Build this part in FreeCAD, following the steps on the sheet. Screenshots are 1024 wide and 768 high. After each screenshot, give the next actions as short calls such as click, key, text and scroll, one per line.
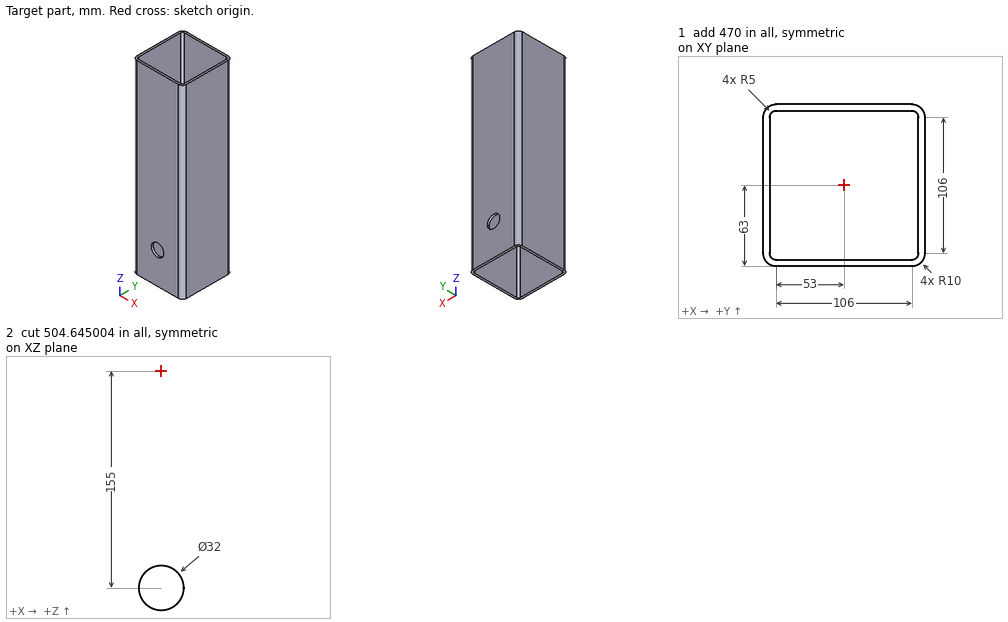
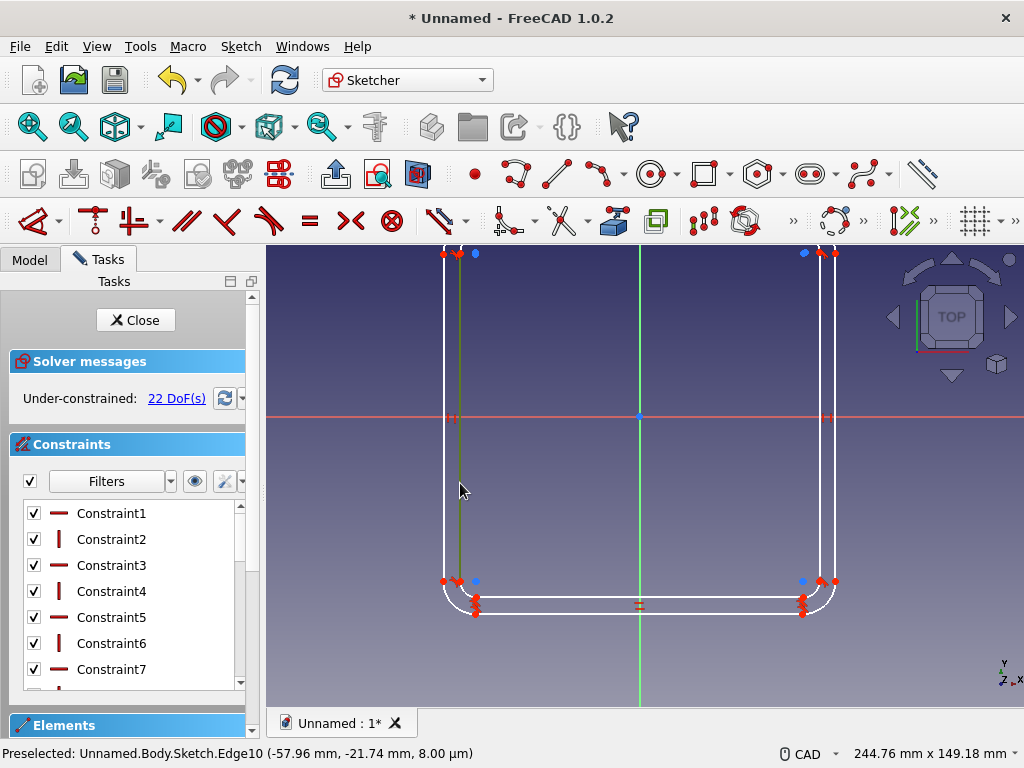
click(465, 593)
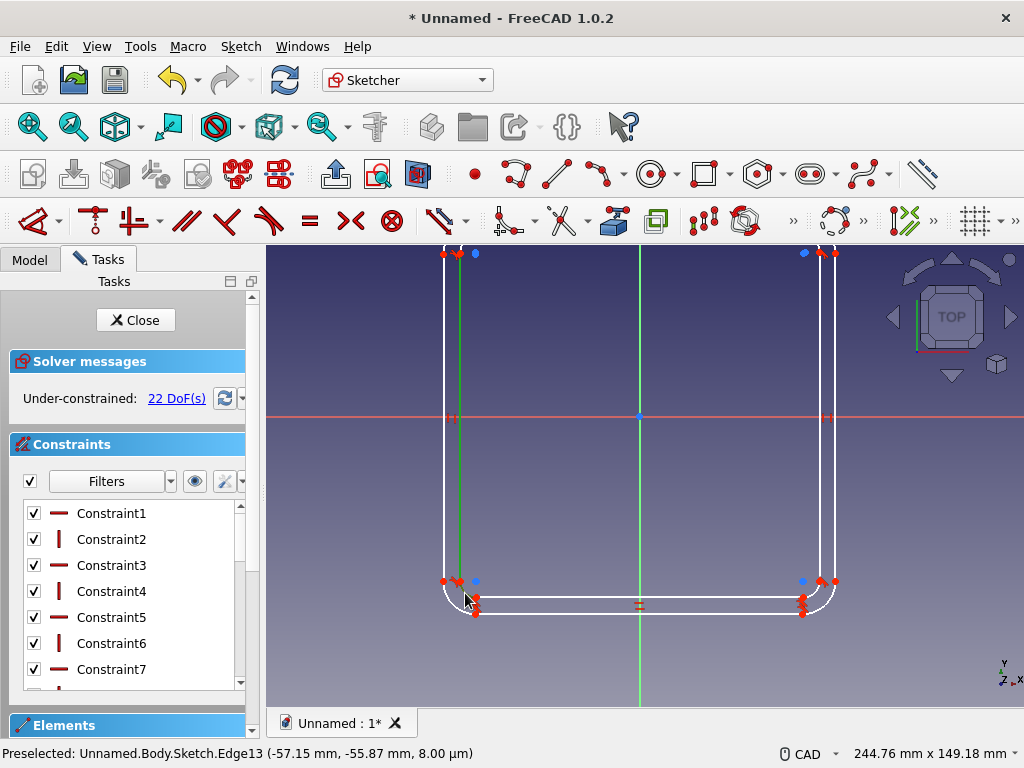
click(269, 222)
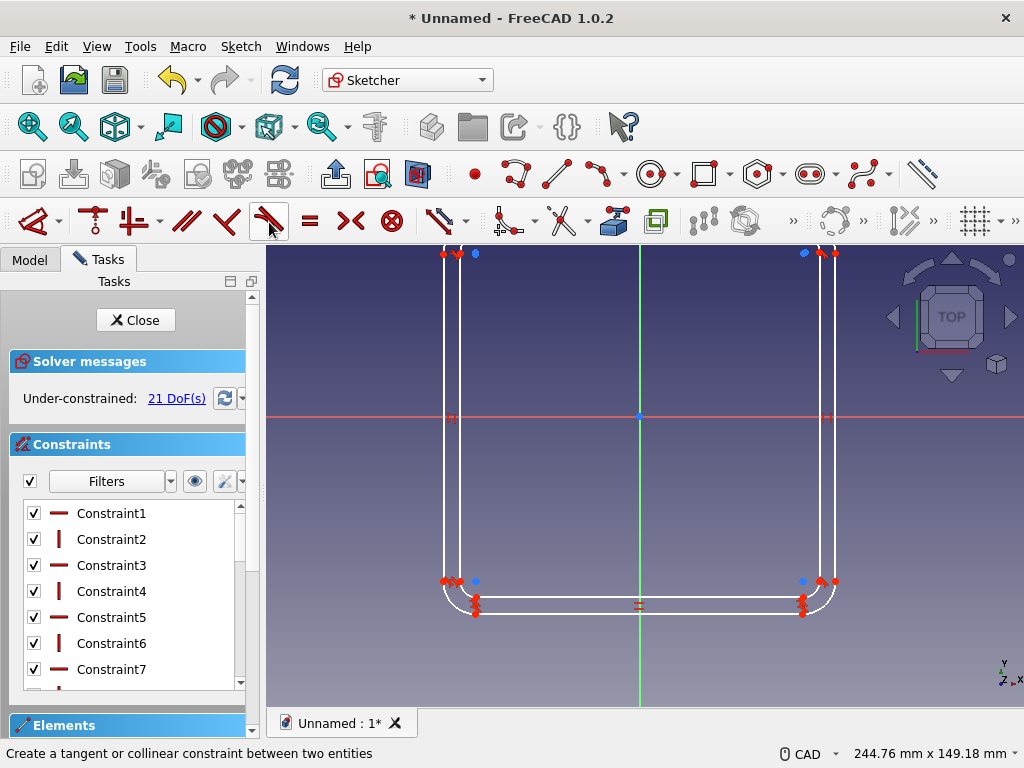
click(460, 483)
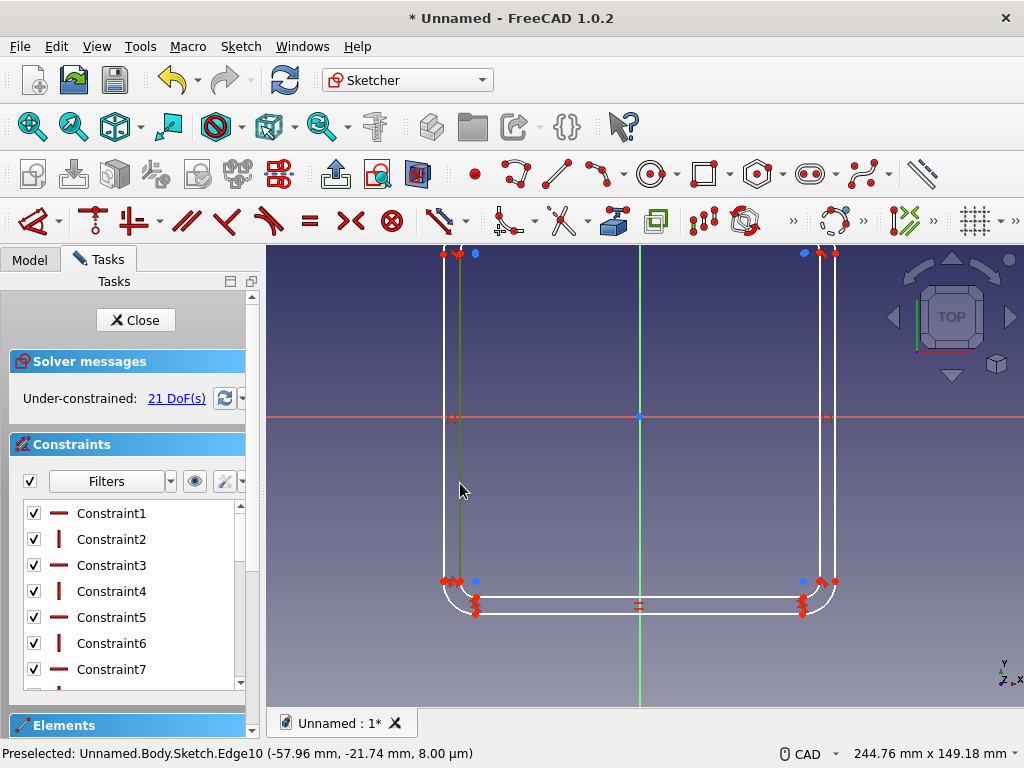
scroll(448, 597, down, 2)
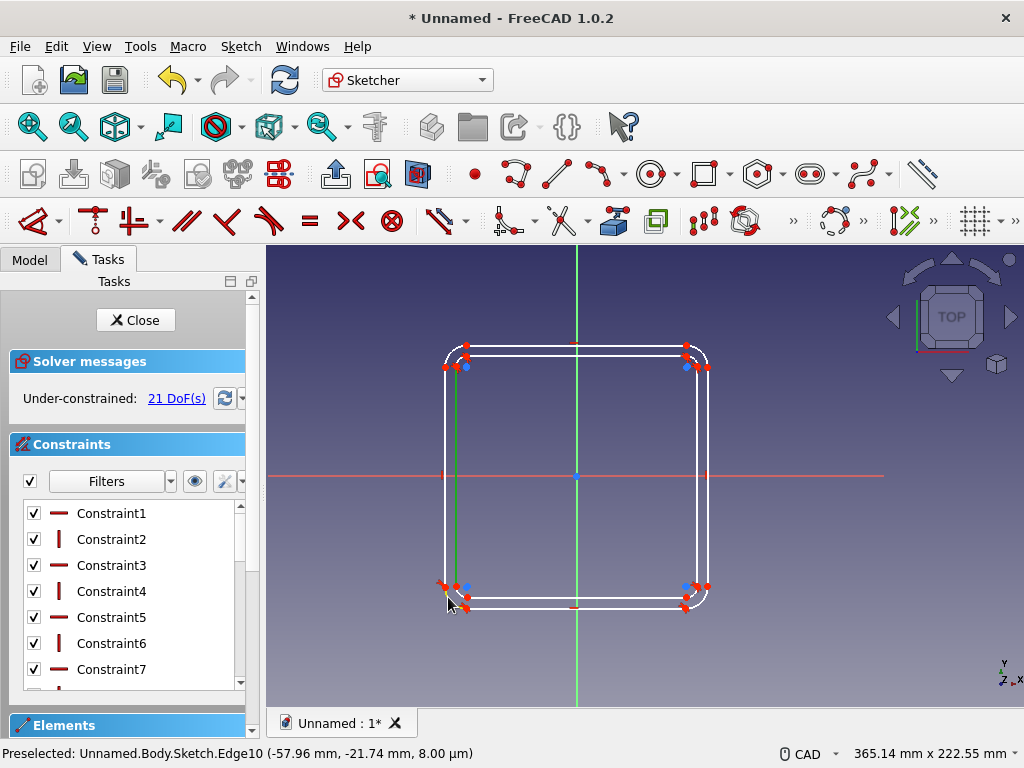
scroll(459, 359, up, 3)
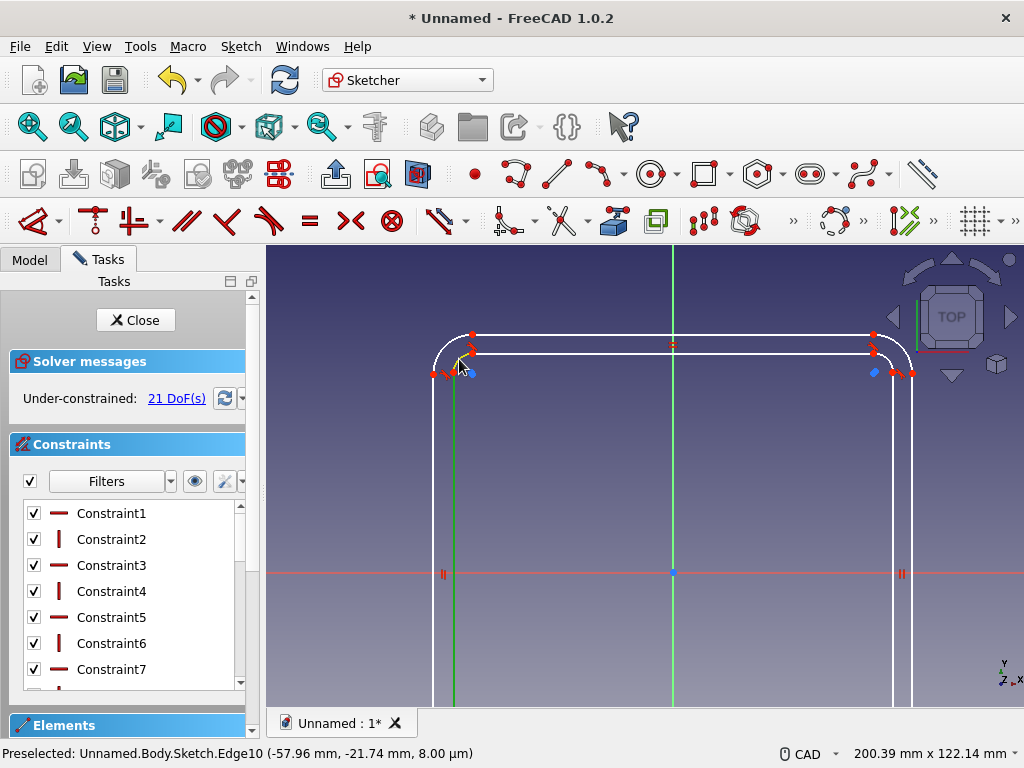
click(459, 359)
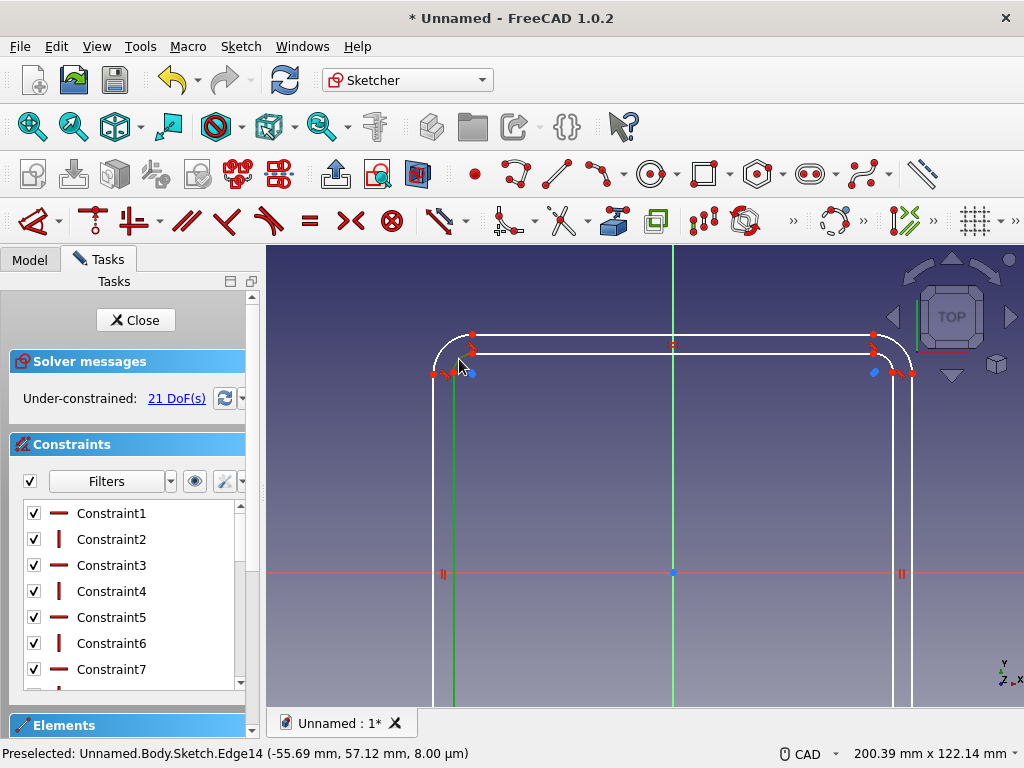
click(269, 222)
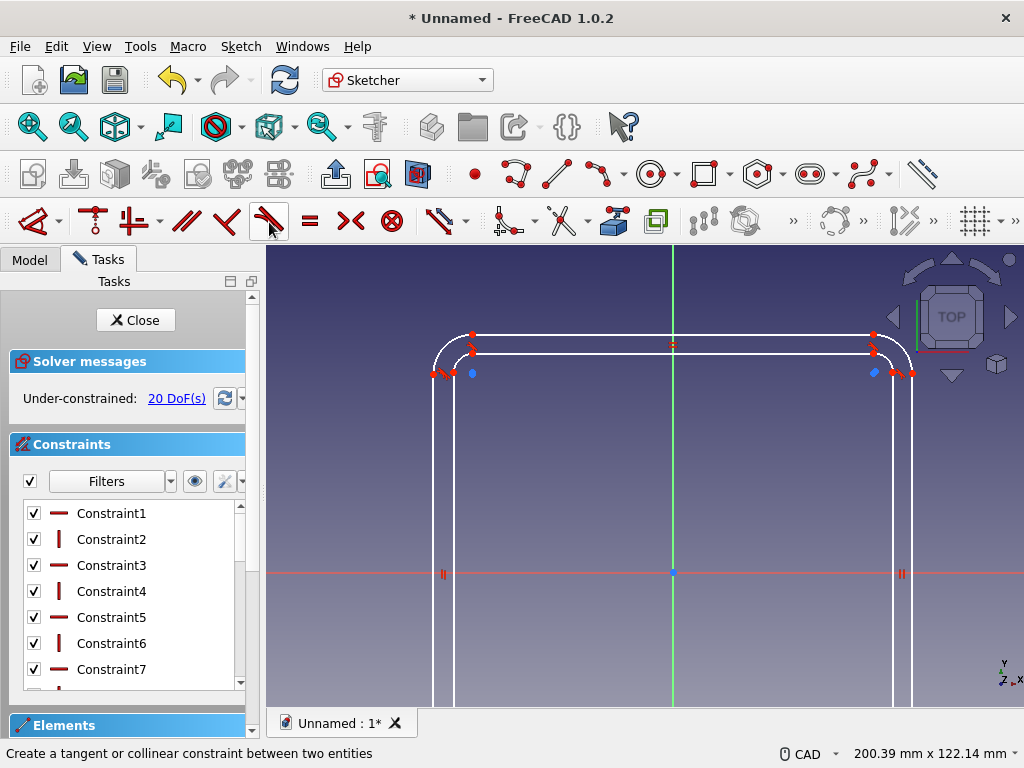
click(593, 354)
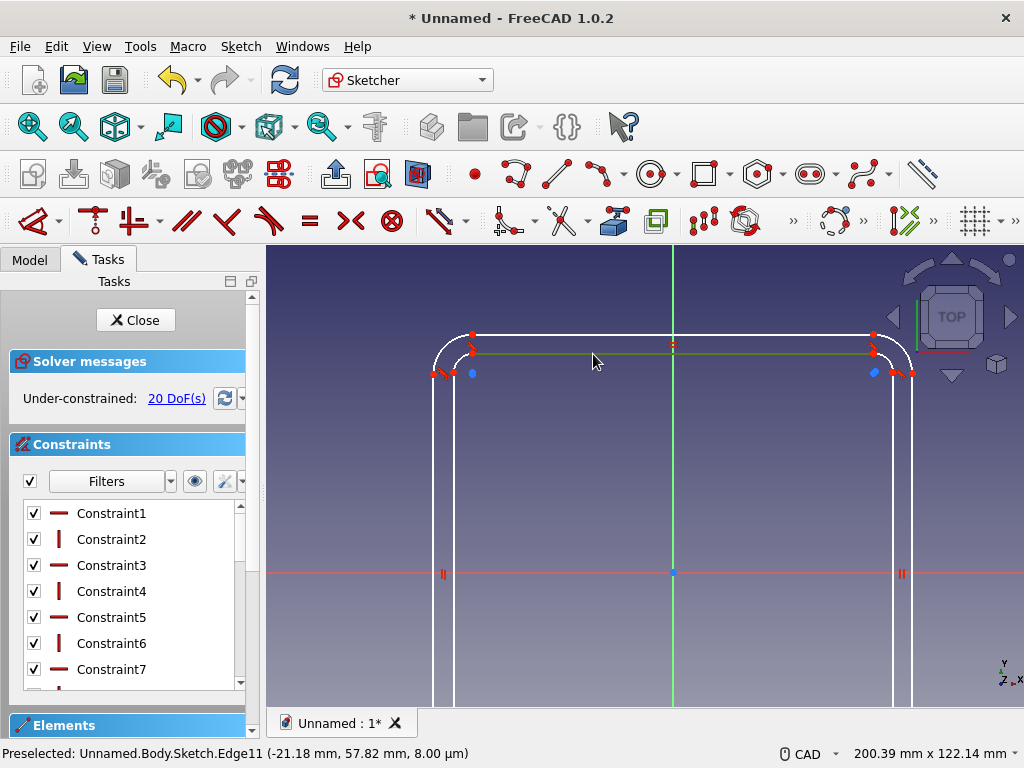
click(459, 360)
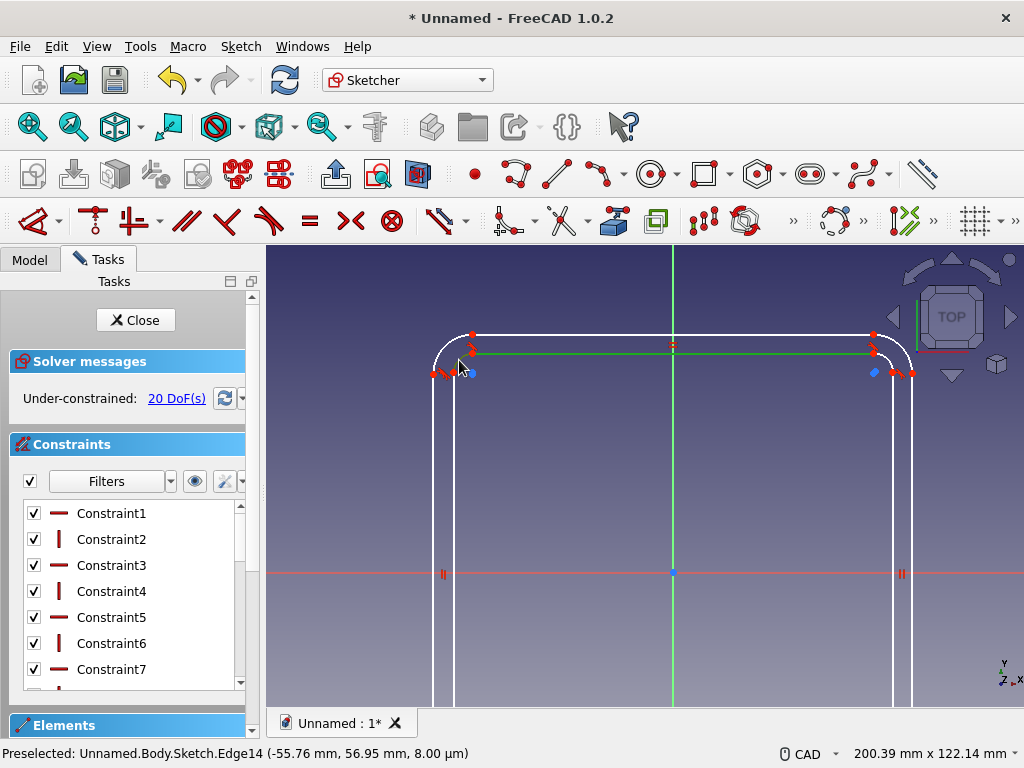
click(269, 222)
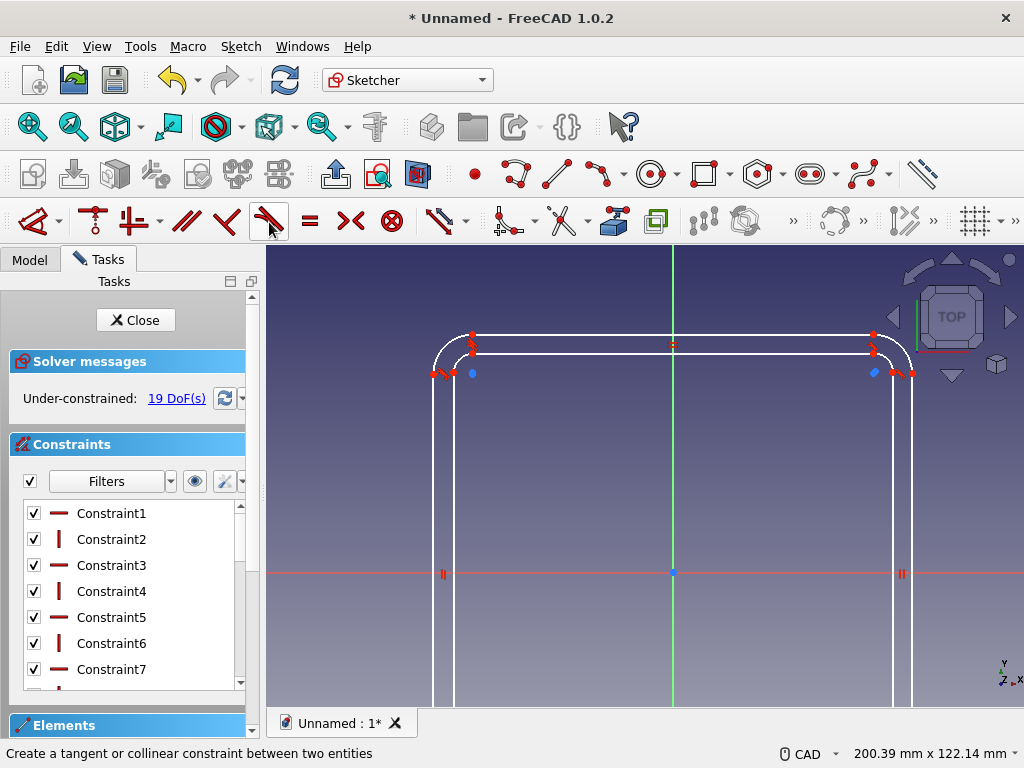
click(593, 354)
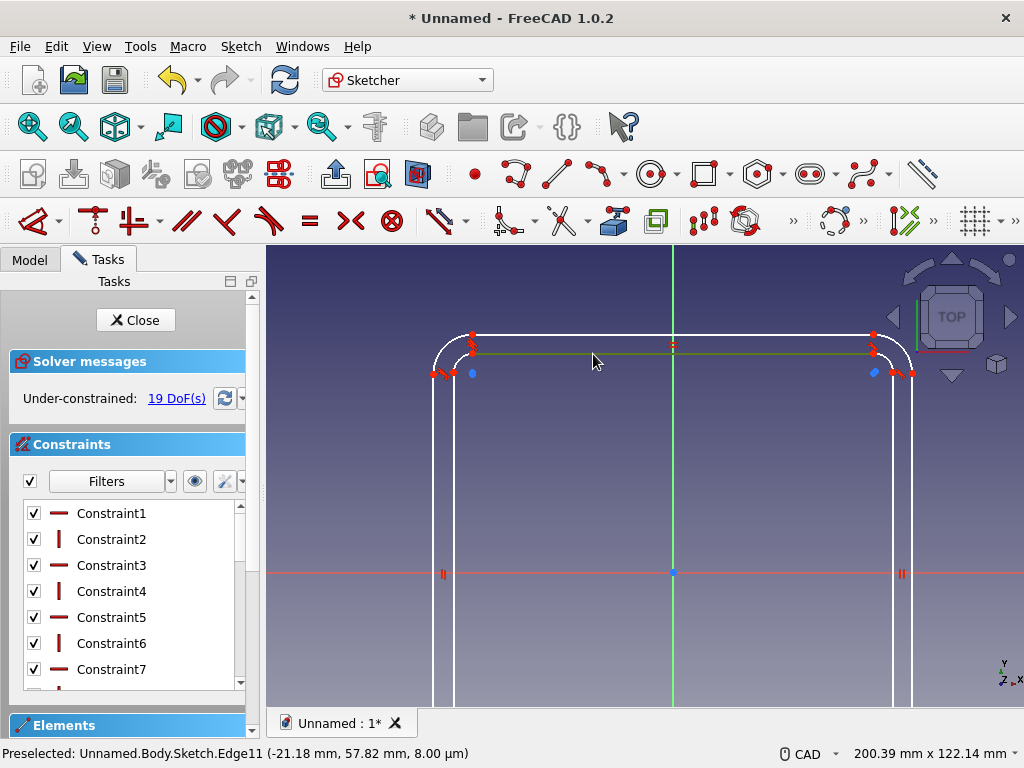
scroll(459, 358, down, 3)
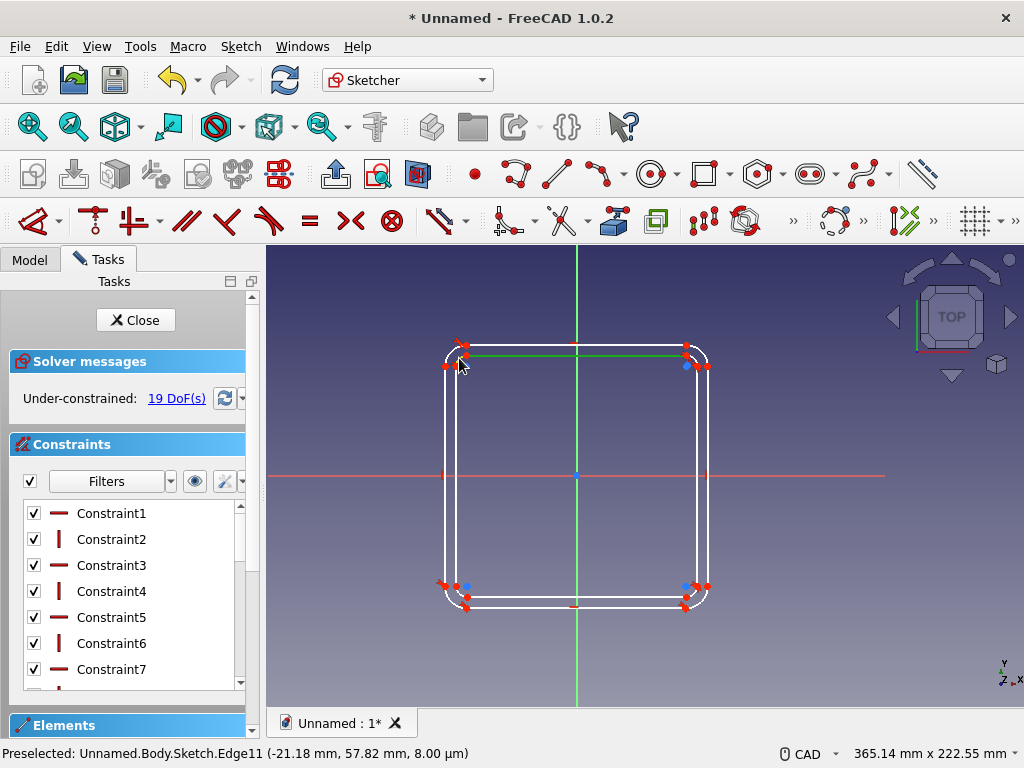
scroll(696, 361, up, 6)